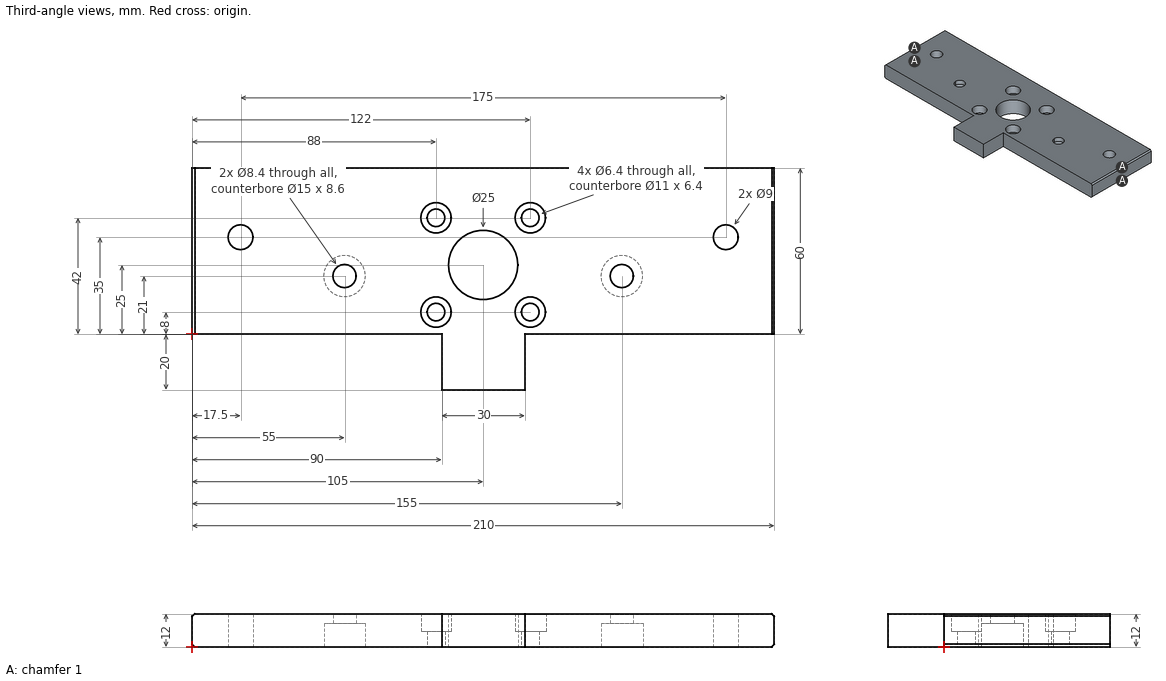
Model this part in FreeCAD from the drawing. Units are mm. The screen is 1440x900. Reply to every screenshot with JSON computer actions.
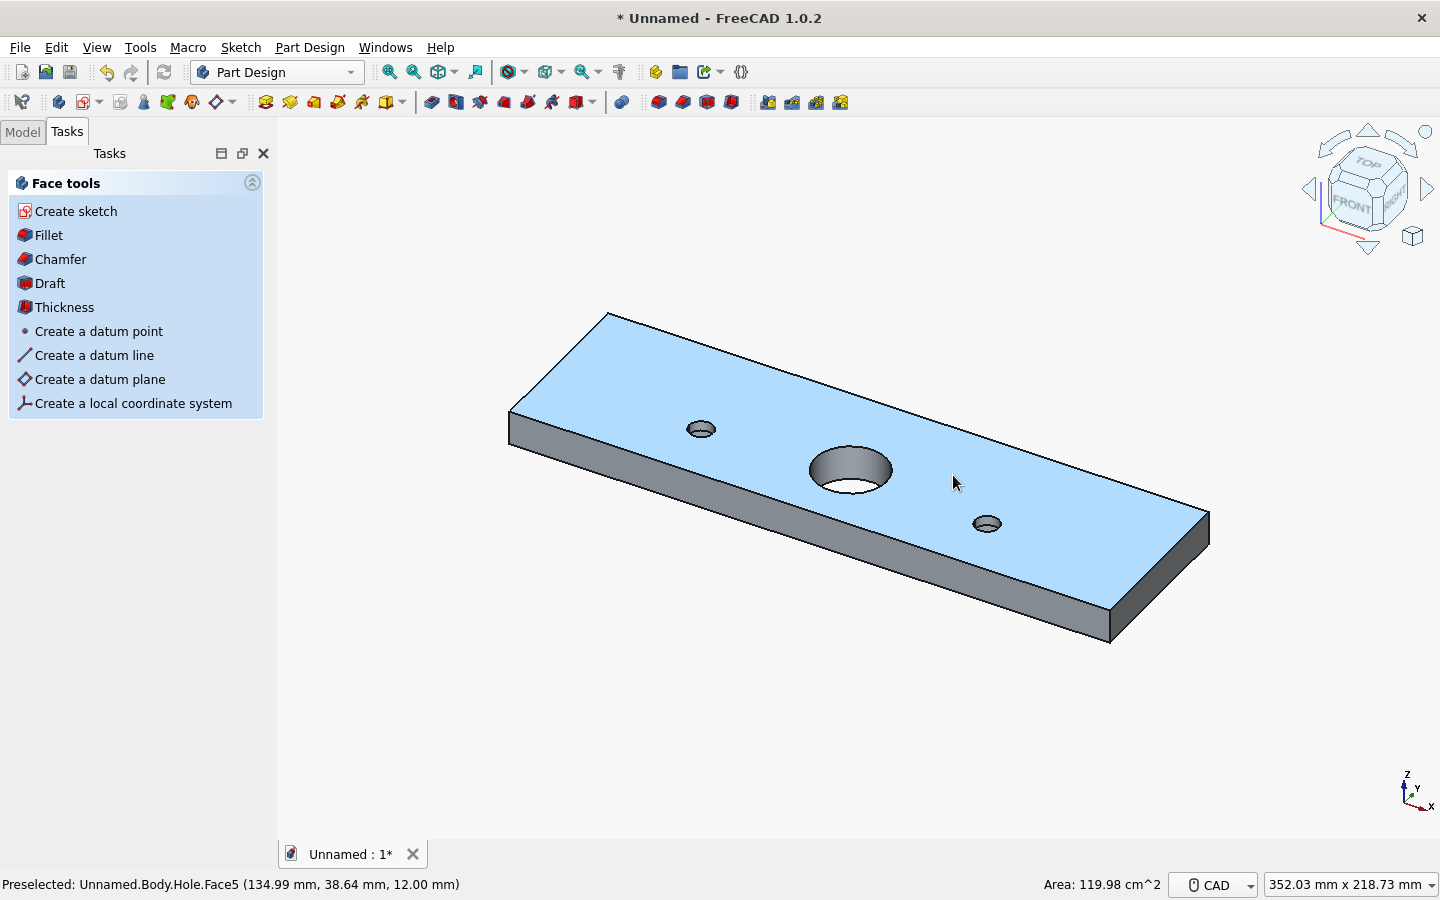
{"action": "left_click", "coordinate": [84, 102]}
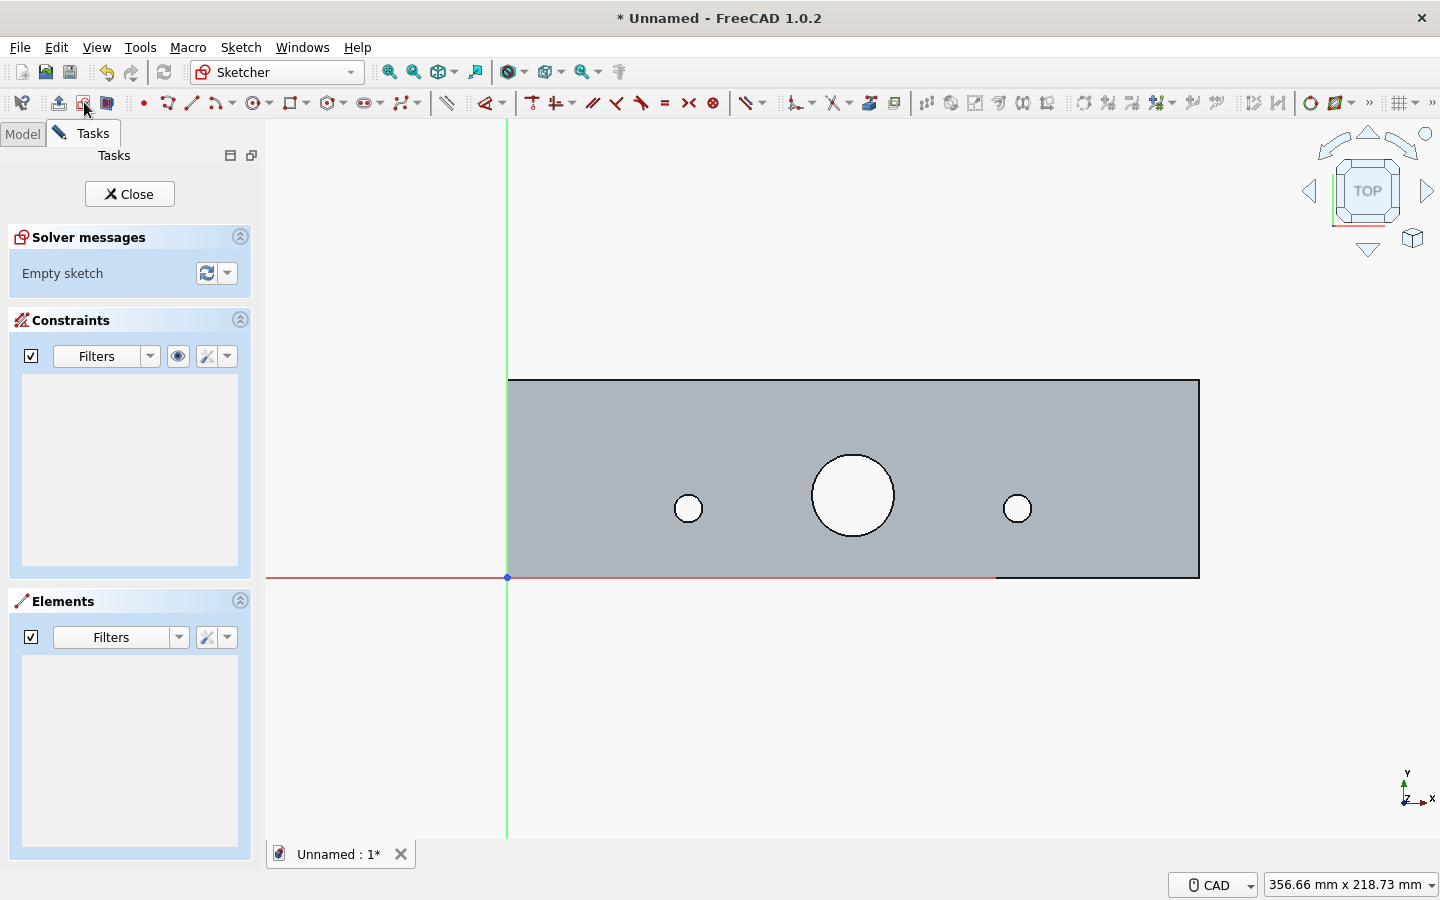
{"action": "scroll", "coordinate": [883, 503], "scroll_direction": "up", "scroll_amount": 6}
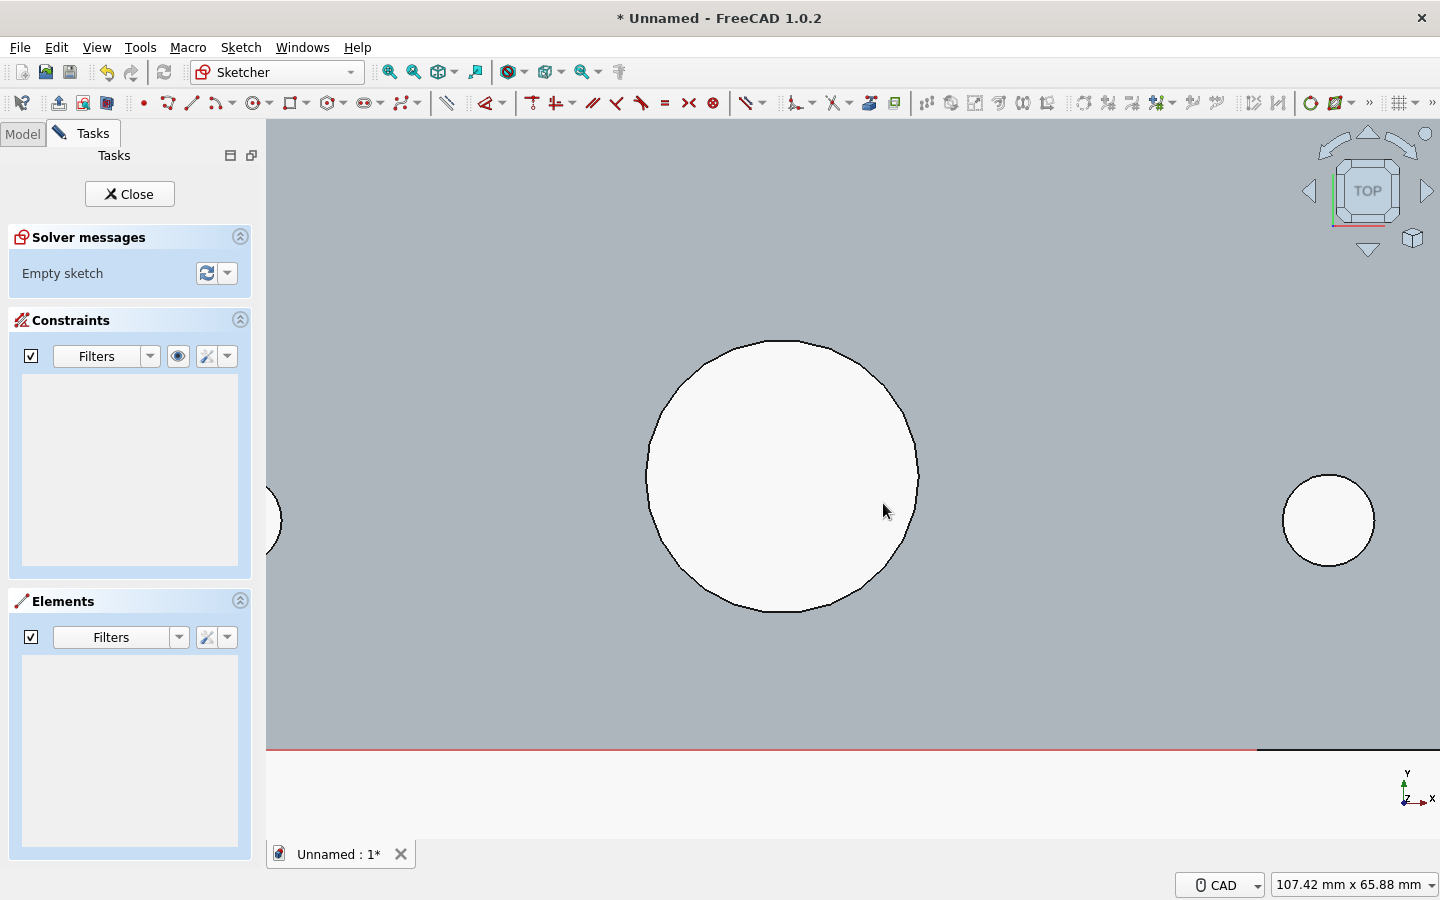
{"action": "key", "text": "g c"}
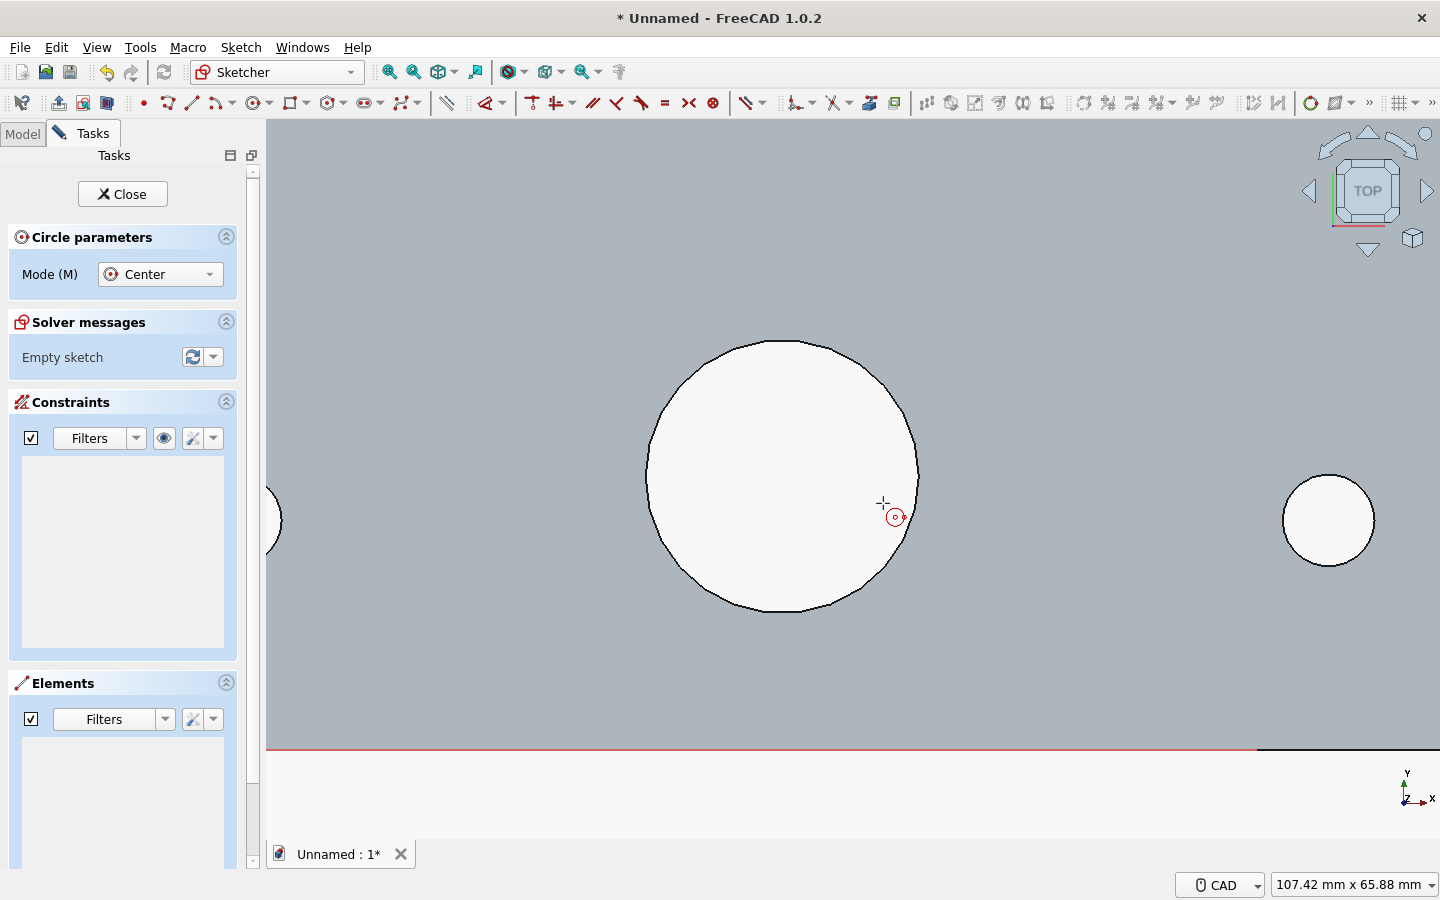
{"action": "left_click", "coordinate": [968, 291]}
{"action": "left_click", "coordinate": [993, 266]}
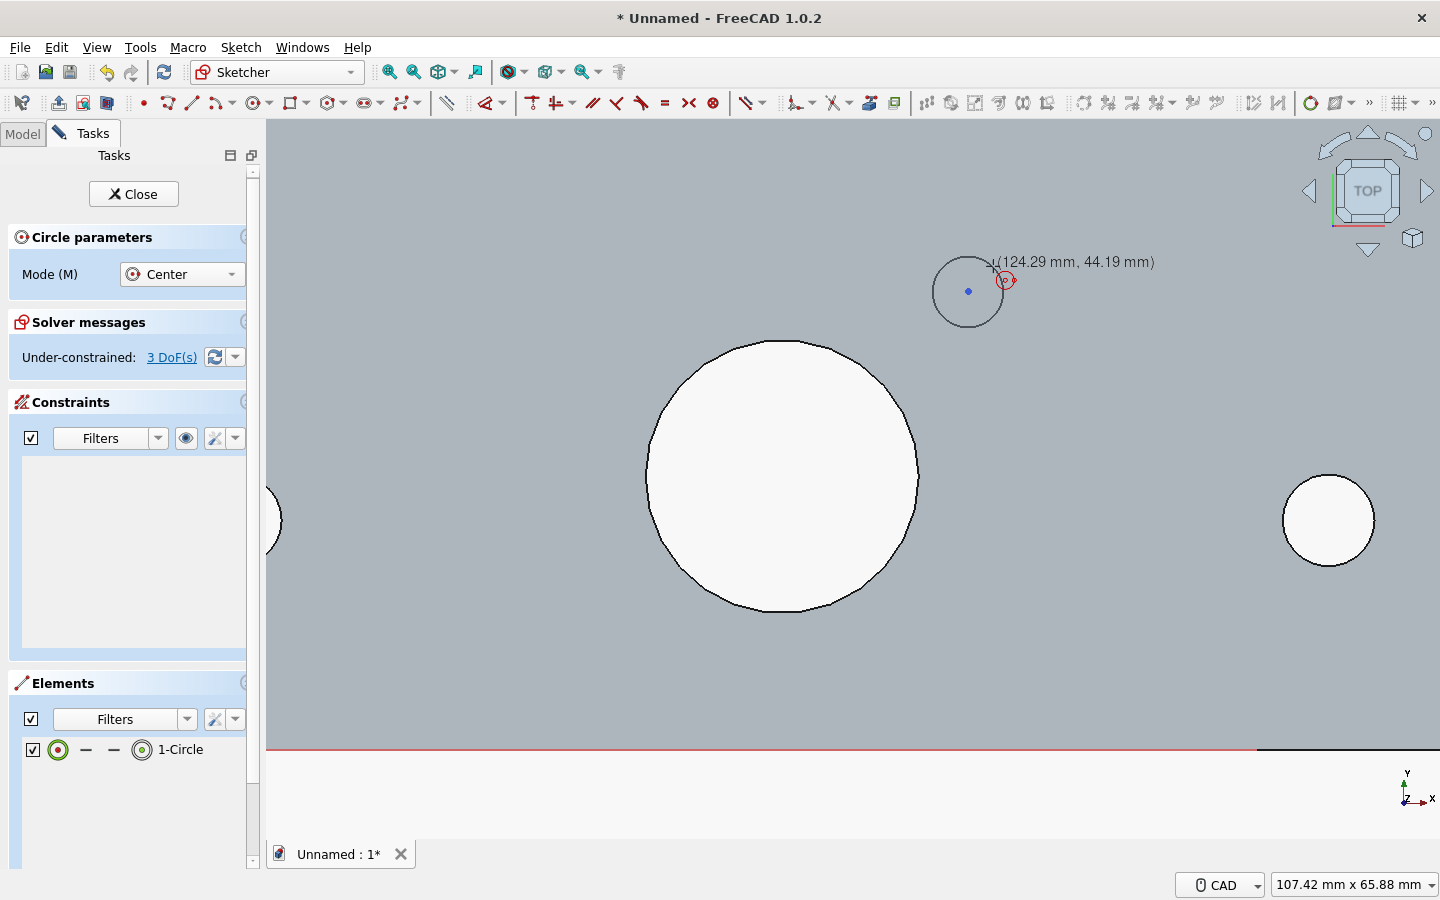
{"action": "left_click", "coordinate": [596, 291]}
{"action": "left_click", "coordinate": [621, 266]}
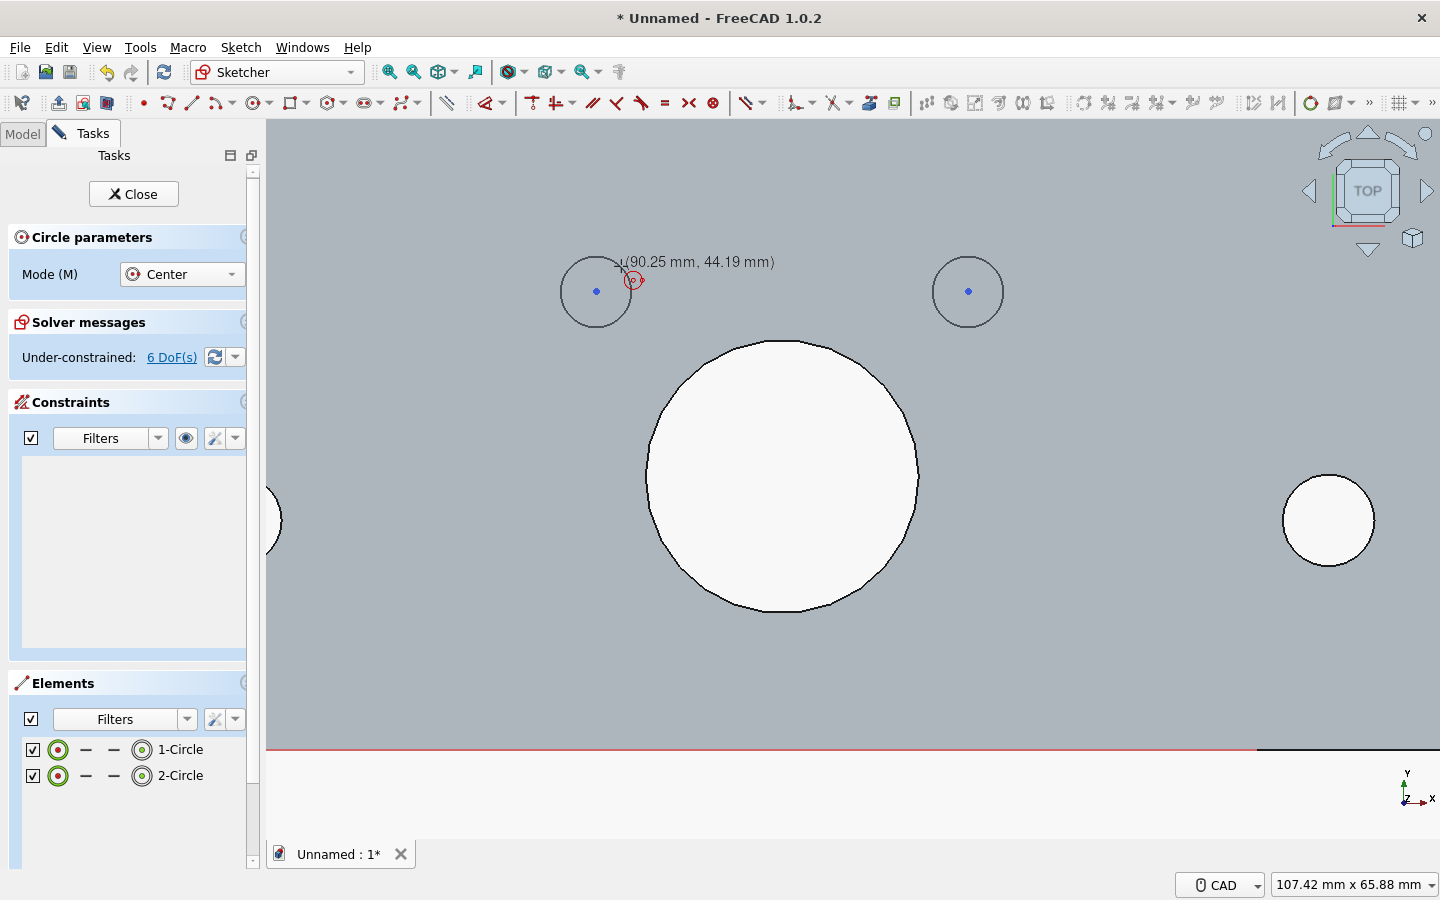
{"action": "left_click", "coordinate": [968, 663]}
{"action": "left_click", "coordinate": [993, 638]}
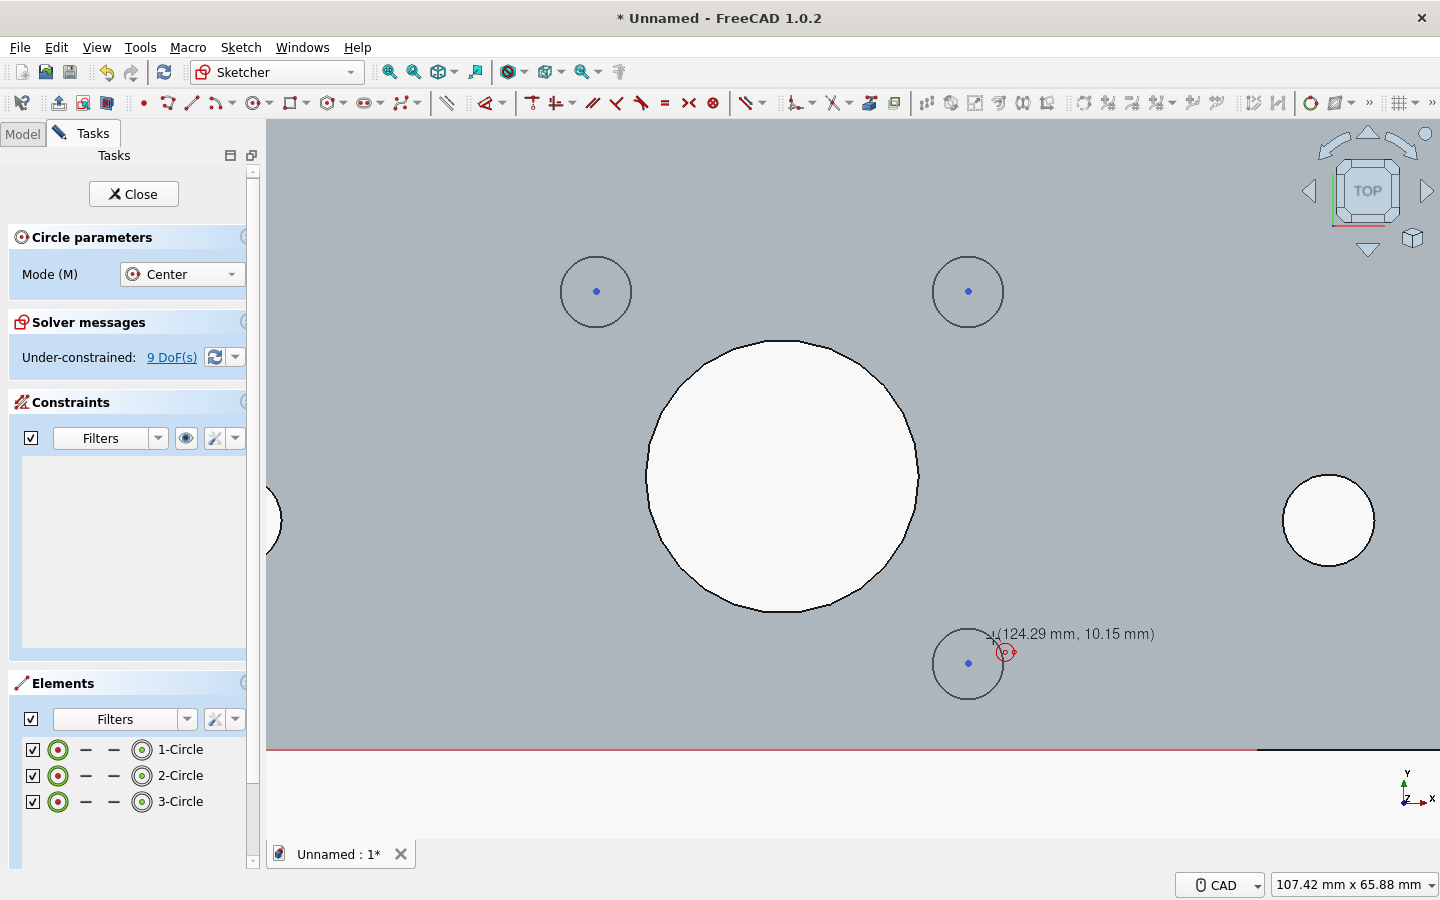
{"action": "left_click", "coordinate": [596, 663]}
{"action": "left_click", "coordinate": [621, 638]}
{"action": "key", "text": "Escape"}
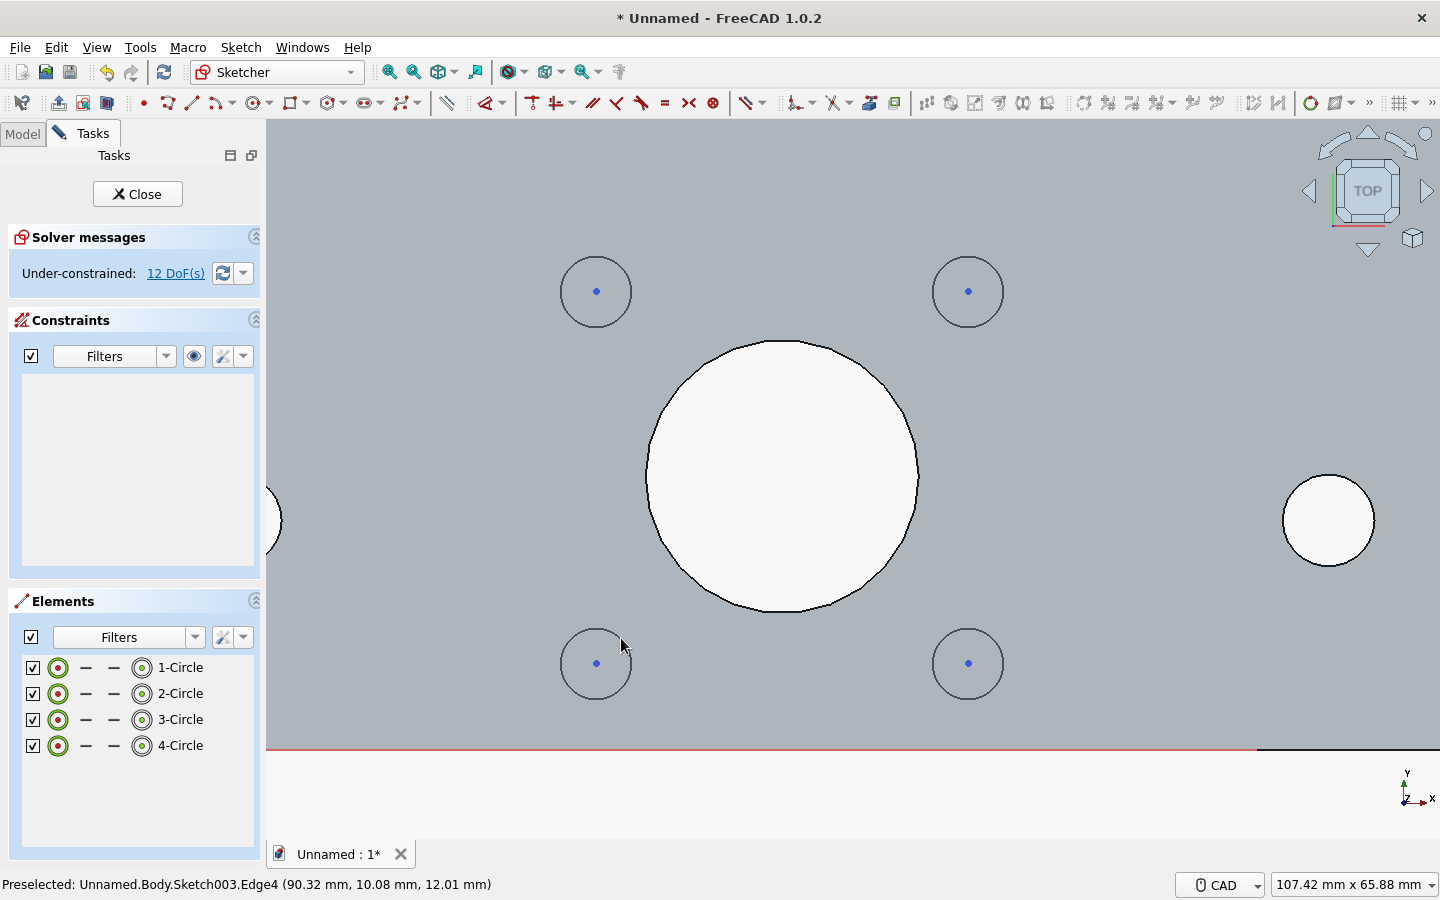
{"action": "left_click", "coordinate": [993, 267]}